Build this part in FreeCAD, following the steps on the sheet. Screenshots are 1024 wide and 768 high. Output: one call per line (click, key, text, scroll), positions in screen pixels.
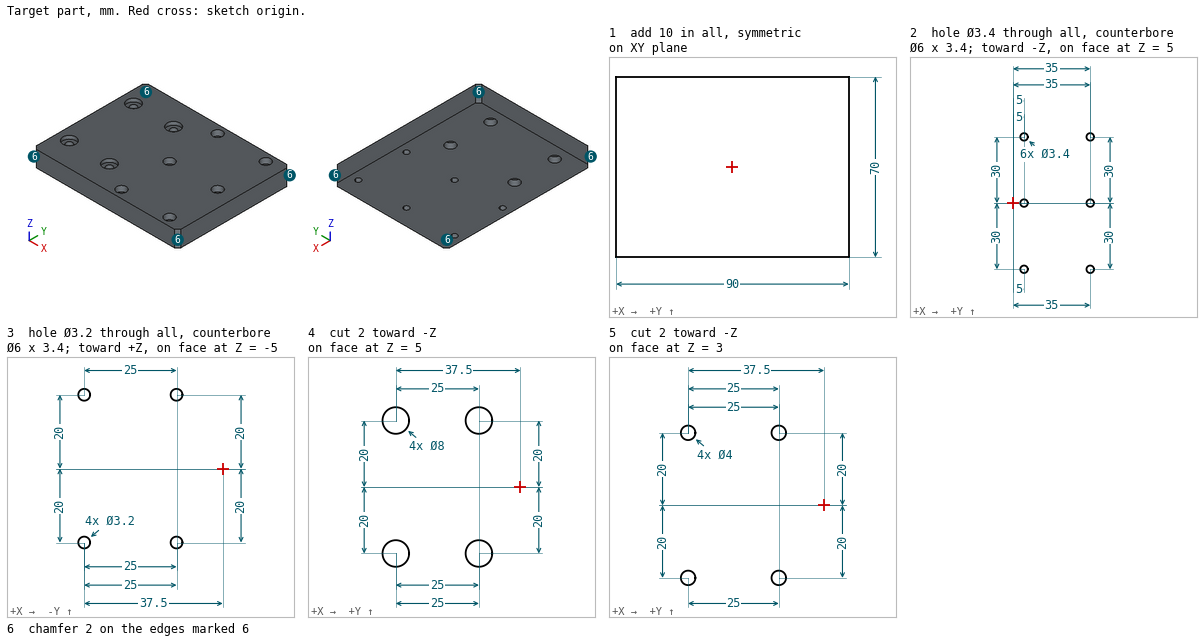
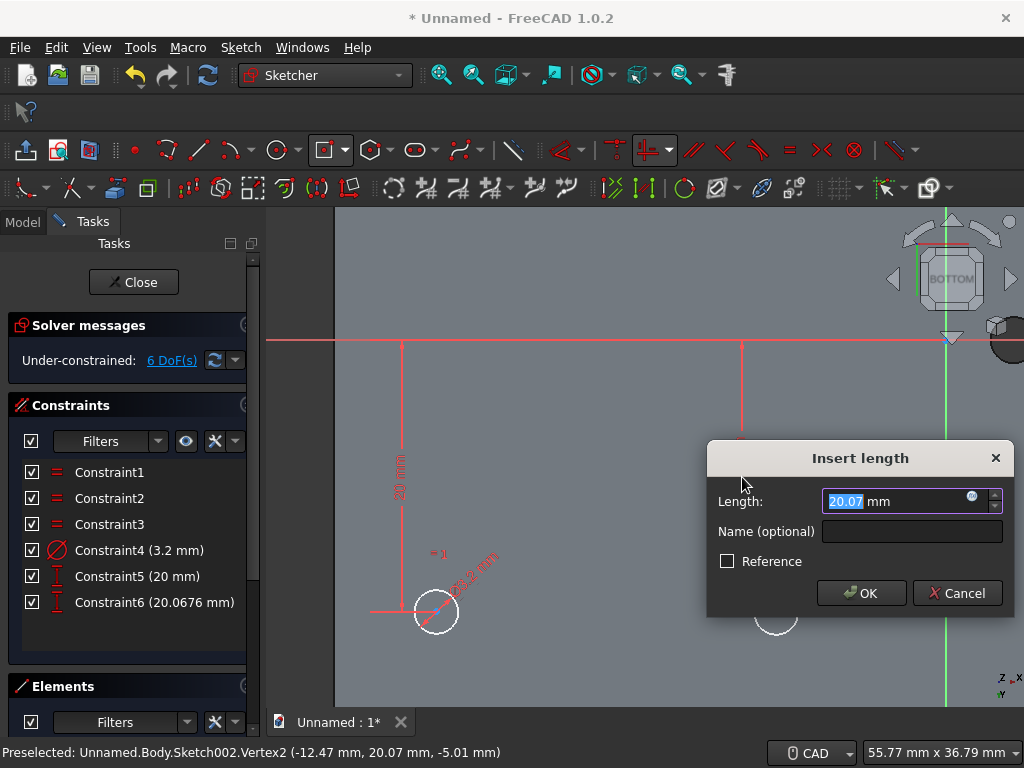
text(20)
key(Return)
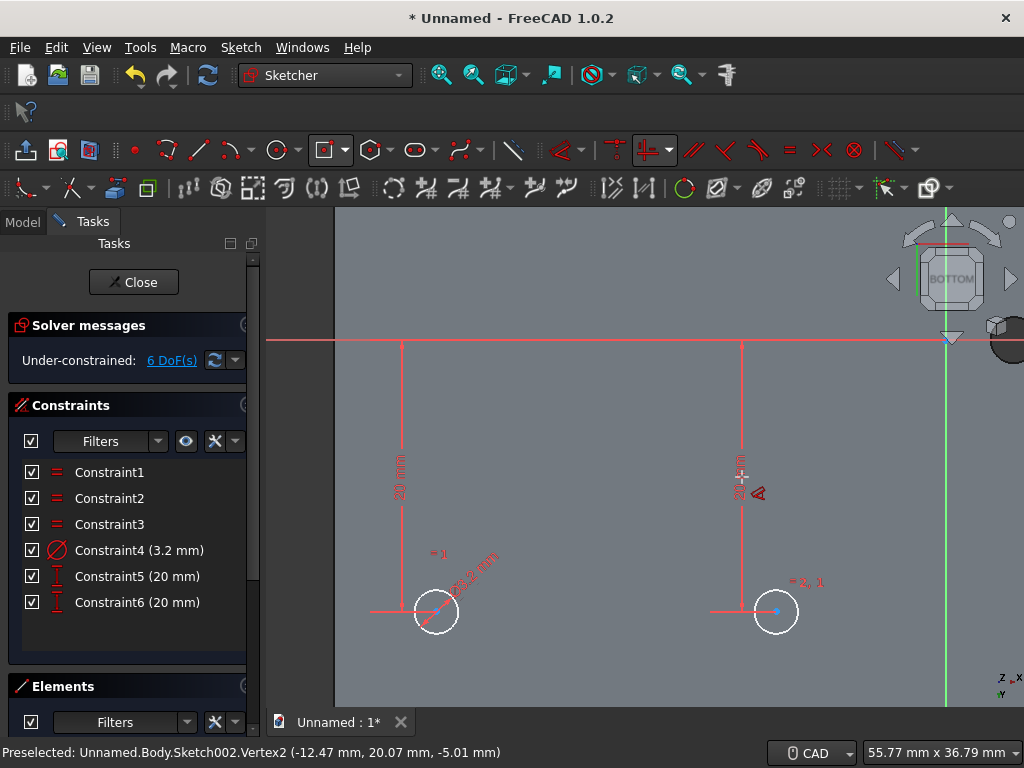
scroll(451, 599, down, 3)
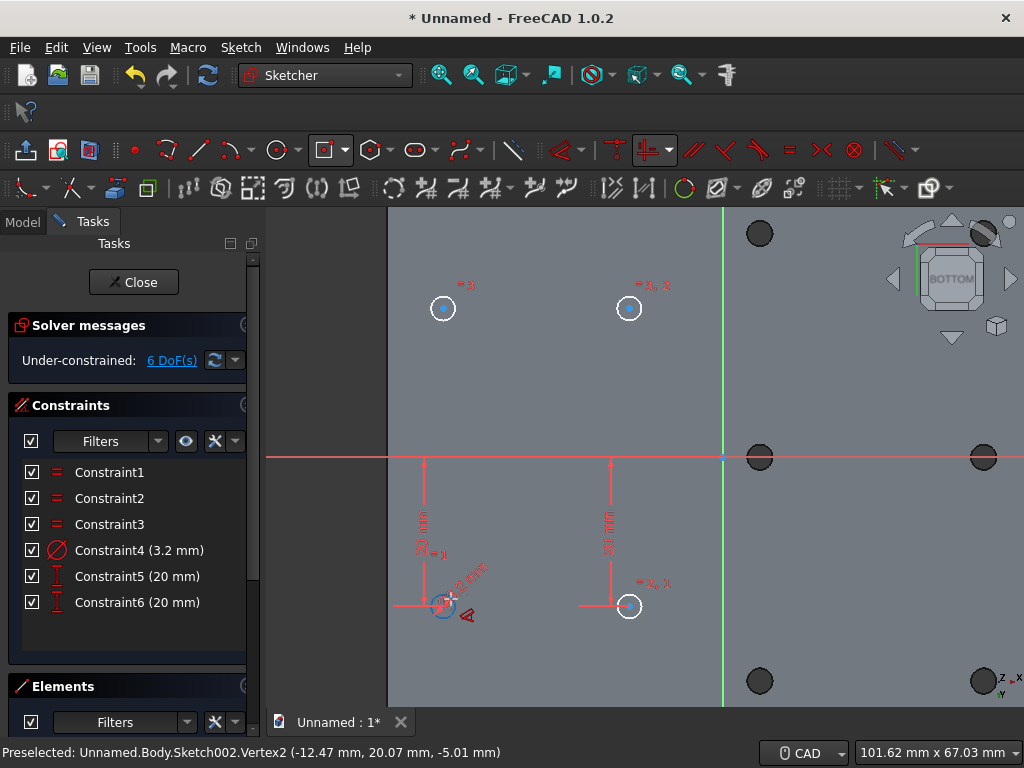
click(629, 309)
click(757, 383)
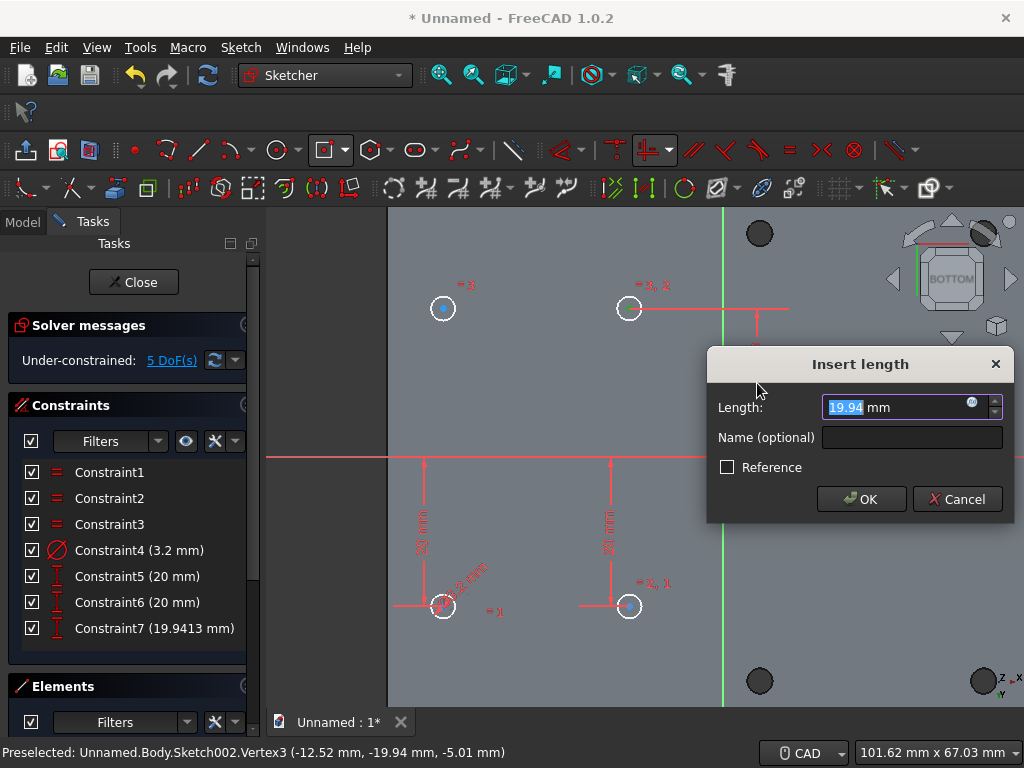
text(20)
key(Return)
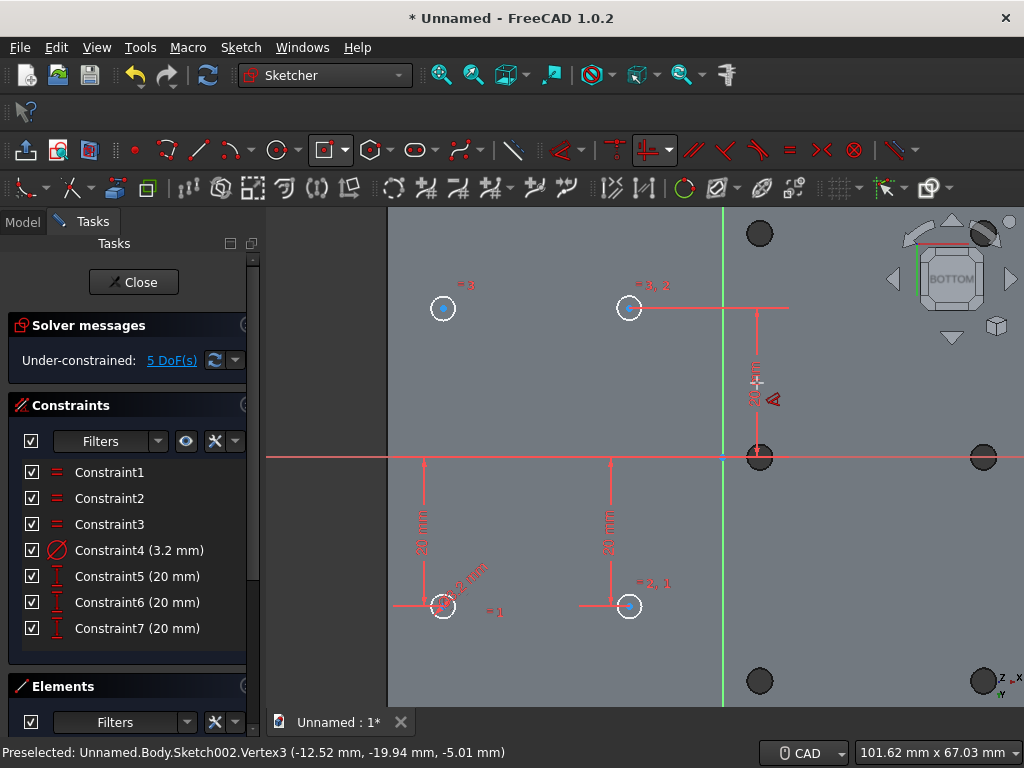
click(443, 309)
click(757, 349)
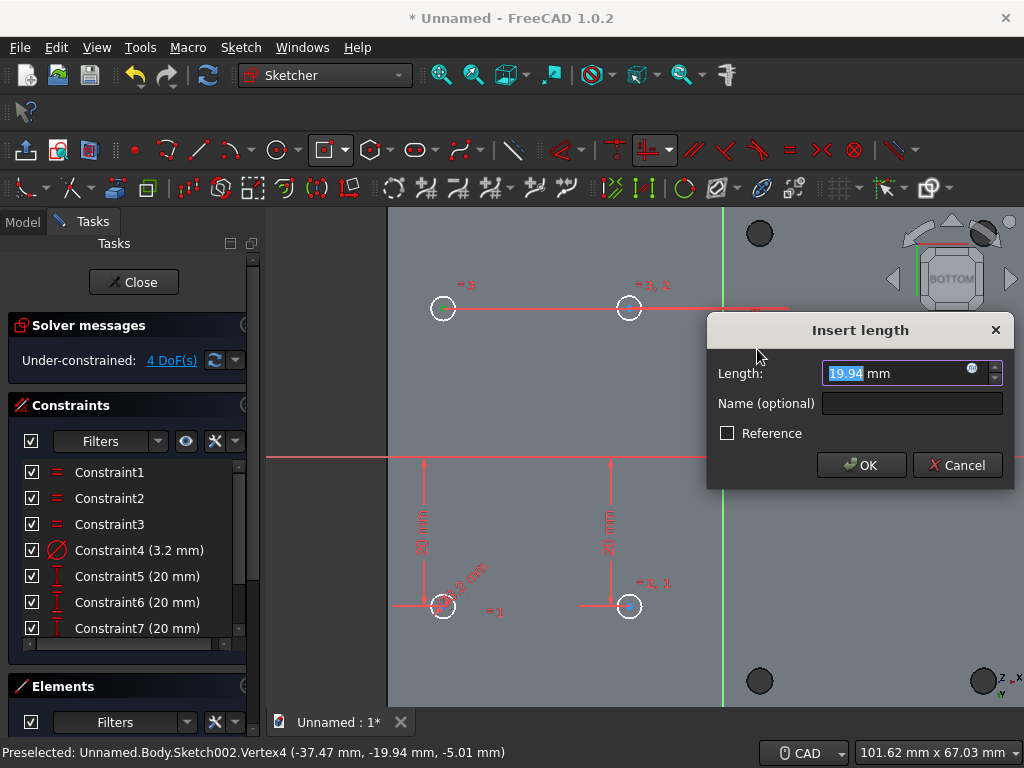
text(20)
key(Return)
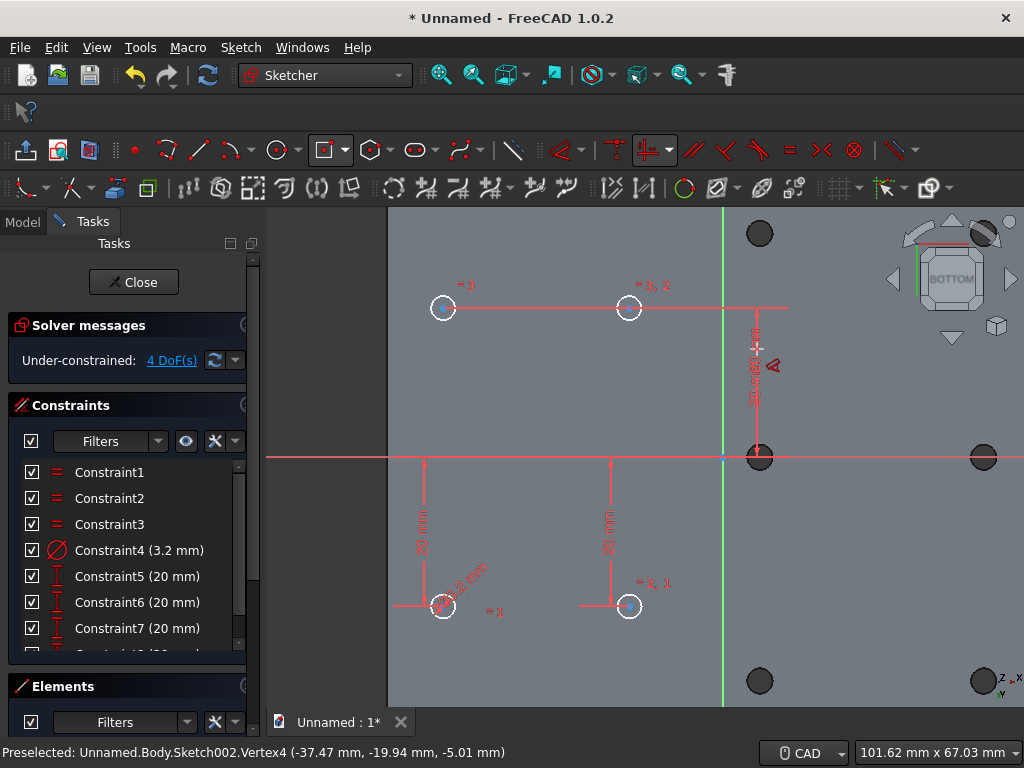
click(443, 606)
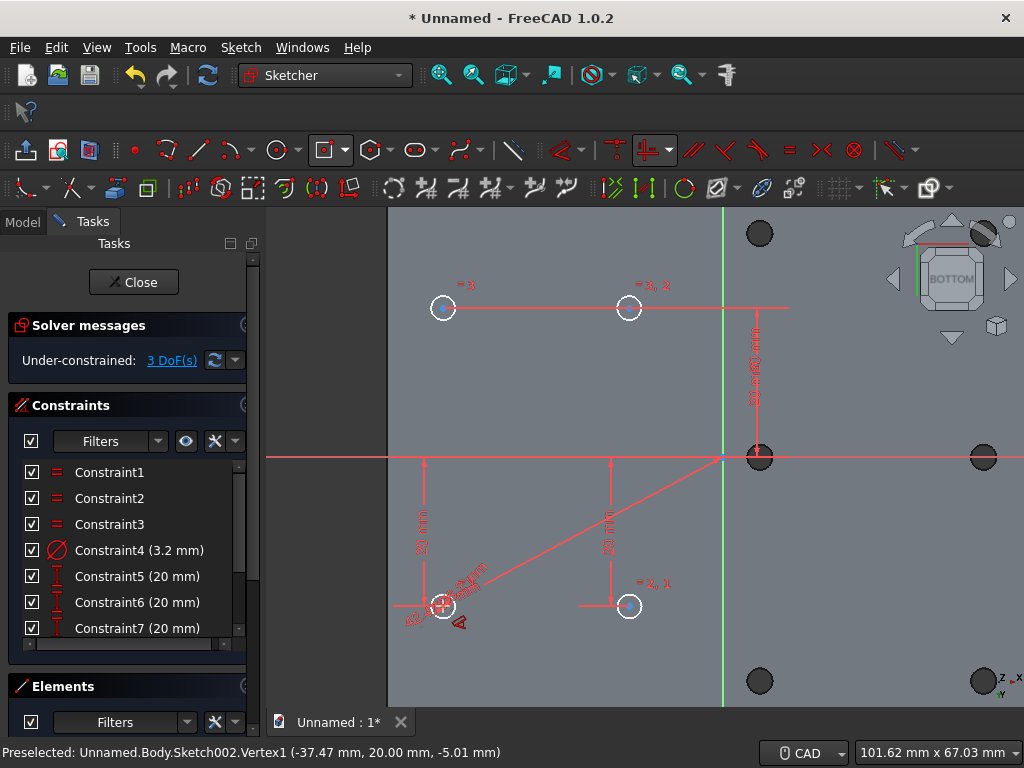
click(630, 606)
click(536, 640)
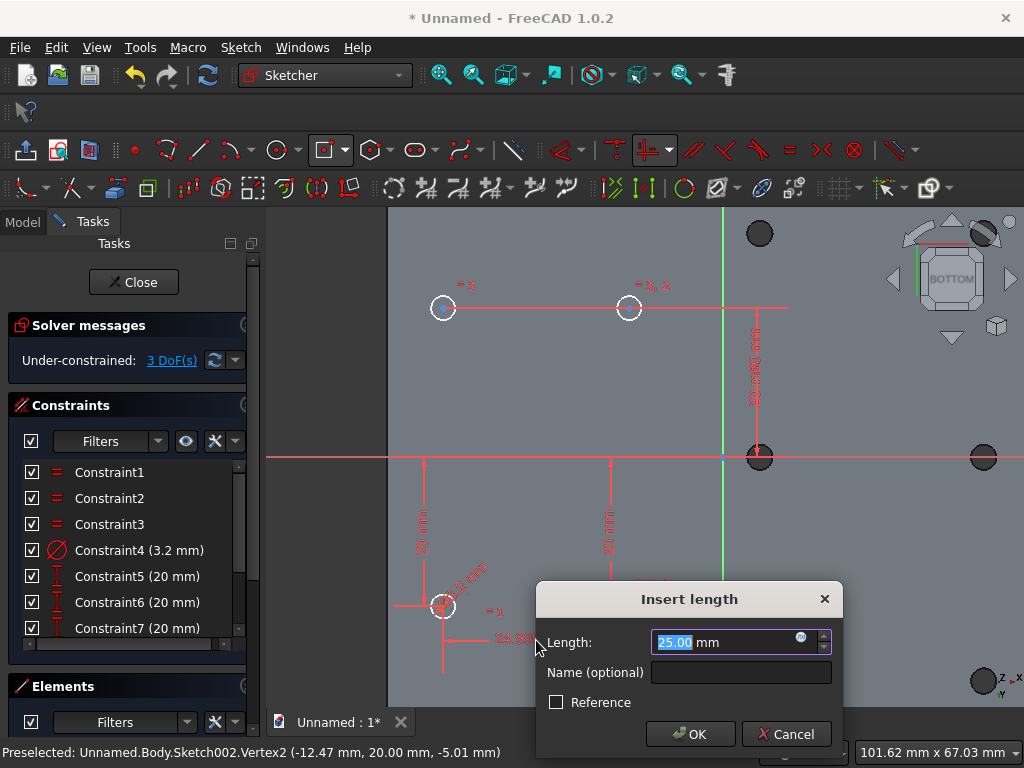
text(25)
key(Return)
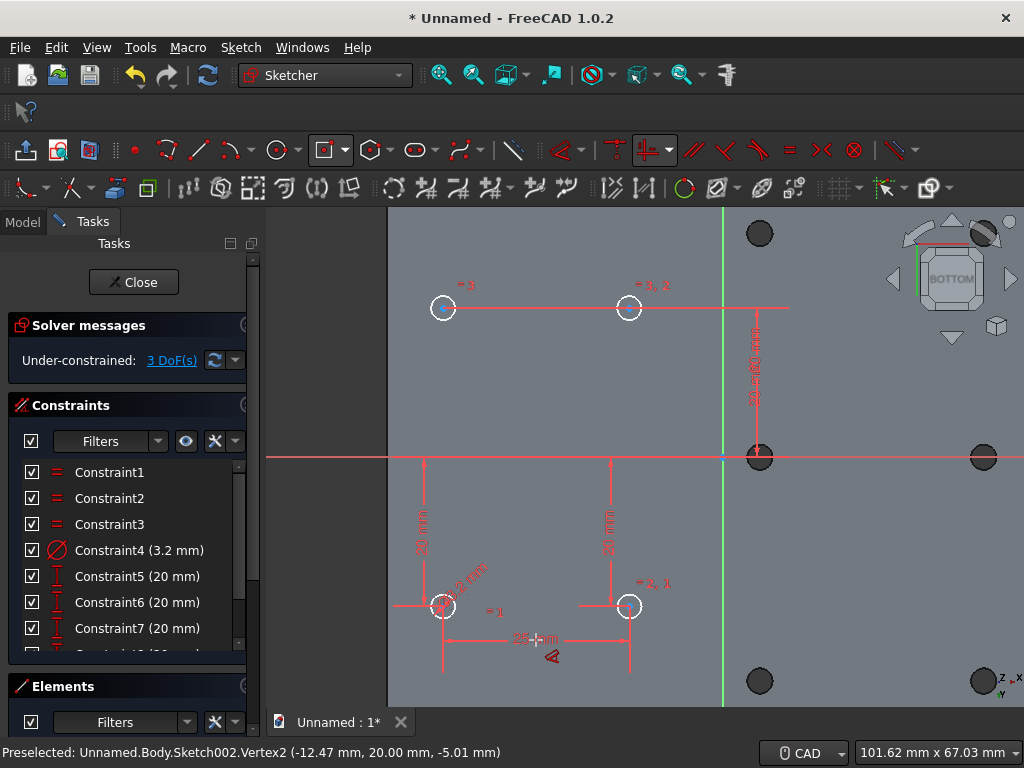
click(443, 606)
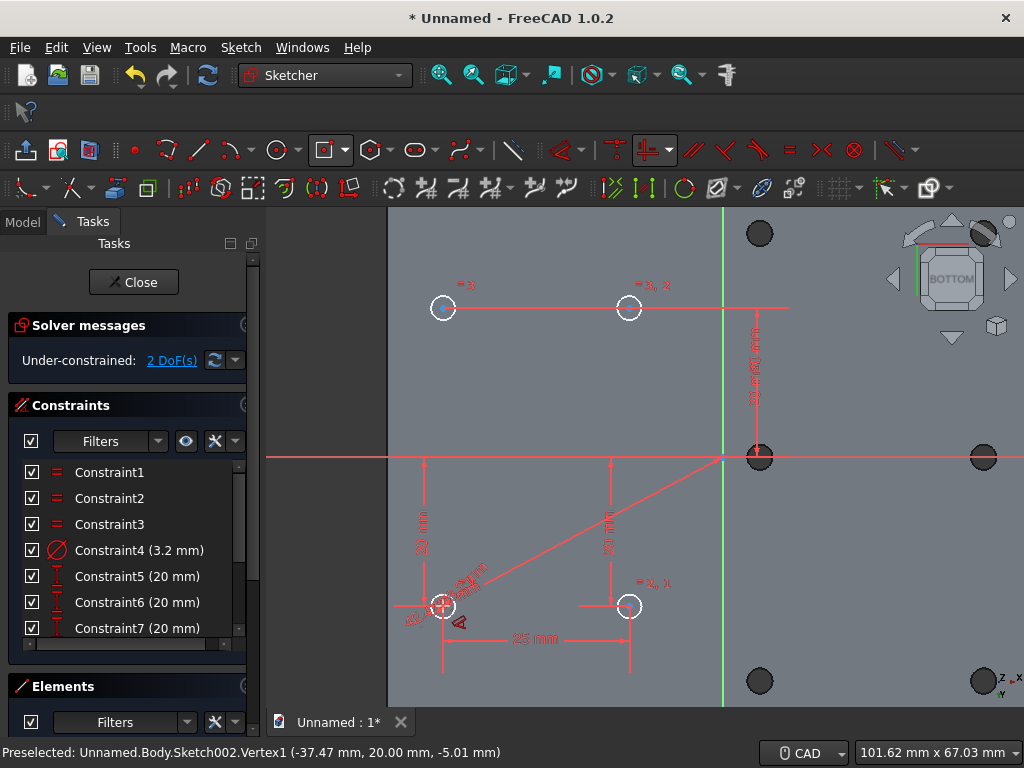
click(629, 308)
click(536, 274)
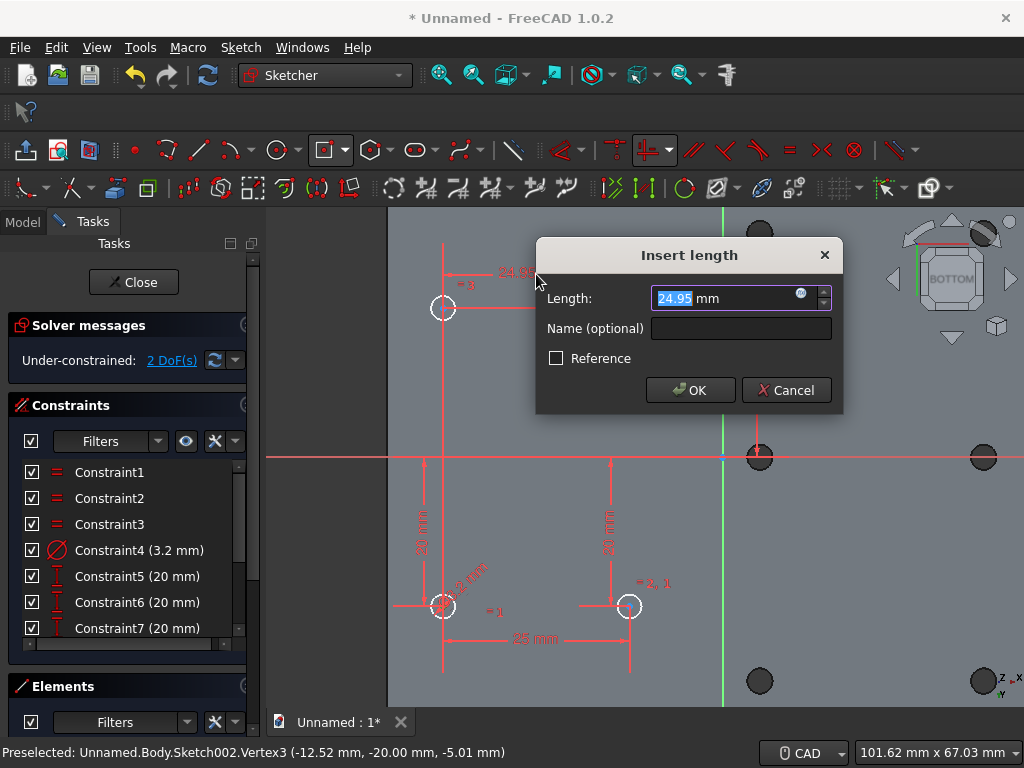
text(25)
key(Return)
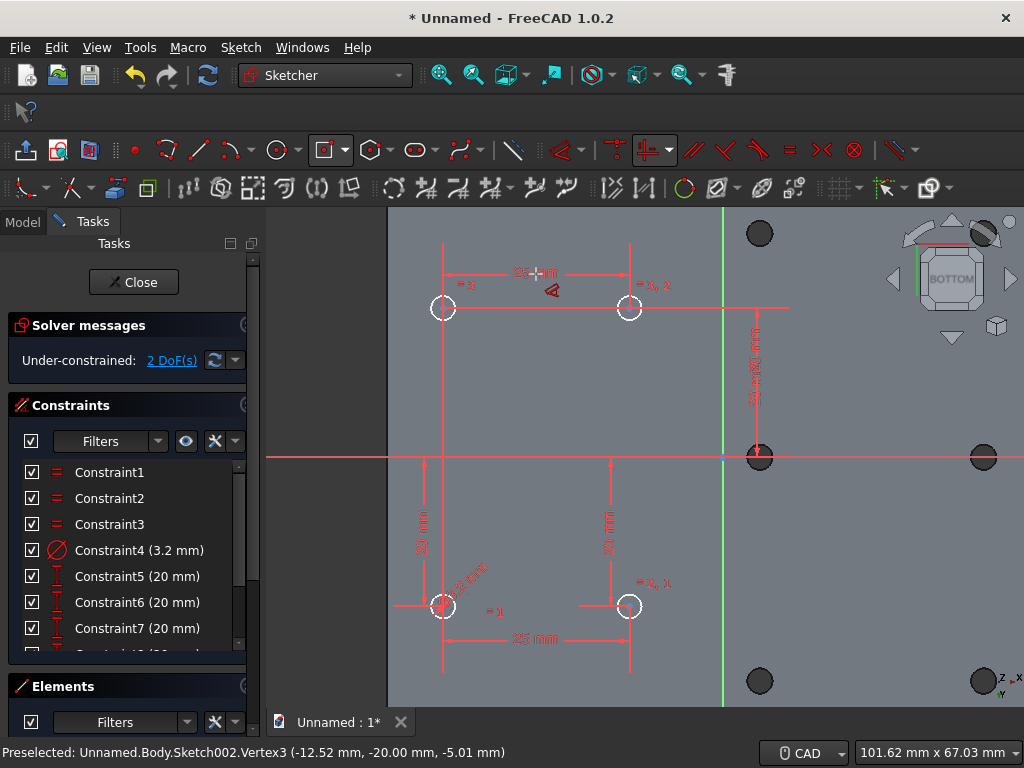
click(630, 308)